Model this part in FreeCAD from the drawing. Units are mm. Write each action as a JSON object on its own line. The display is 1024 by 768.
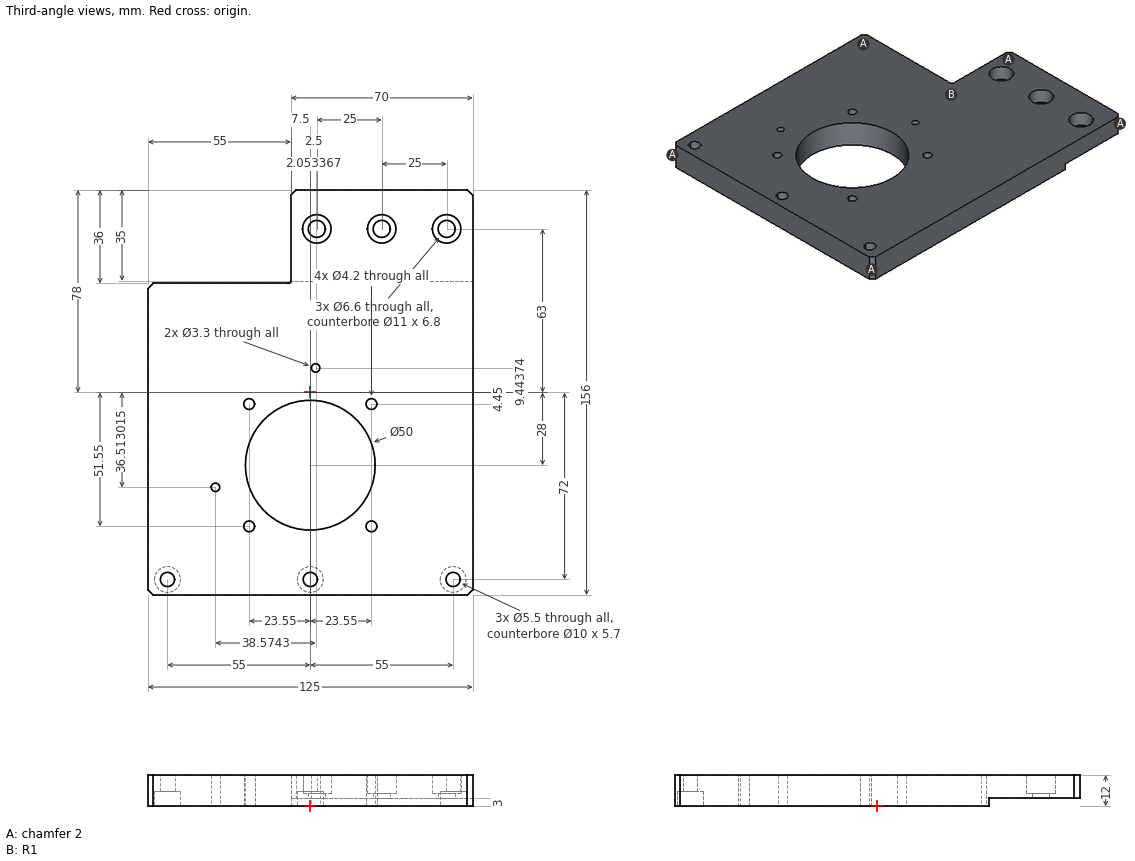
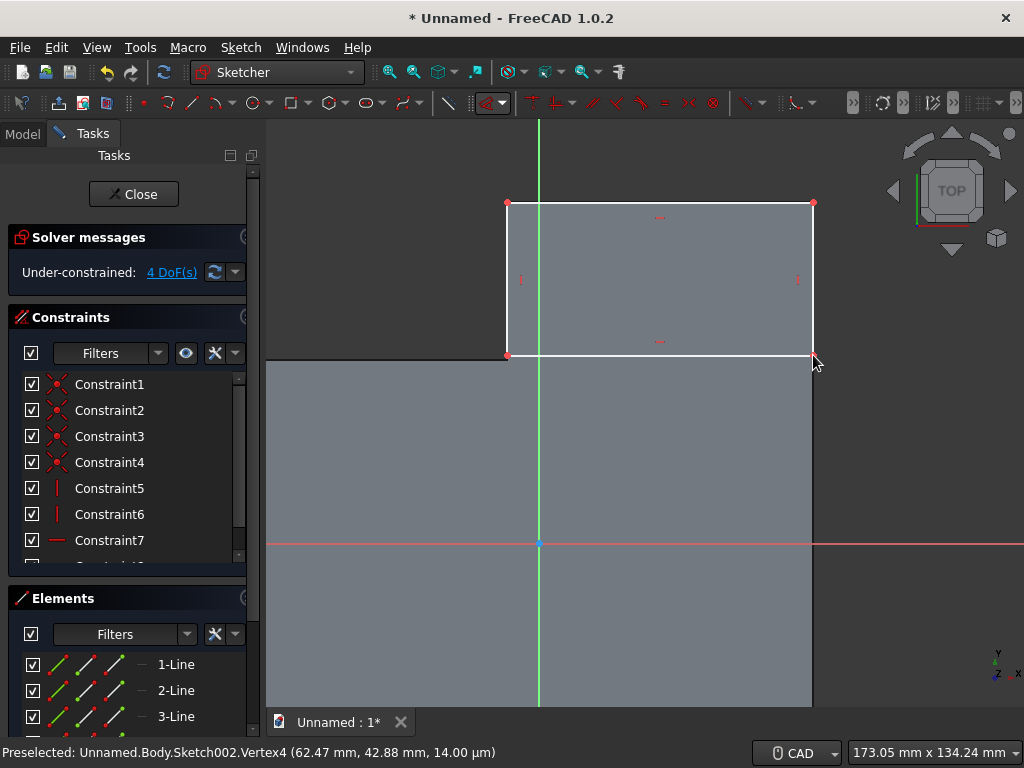
{"action": "left_click", "coordinate": [507, 249]}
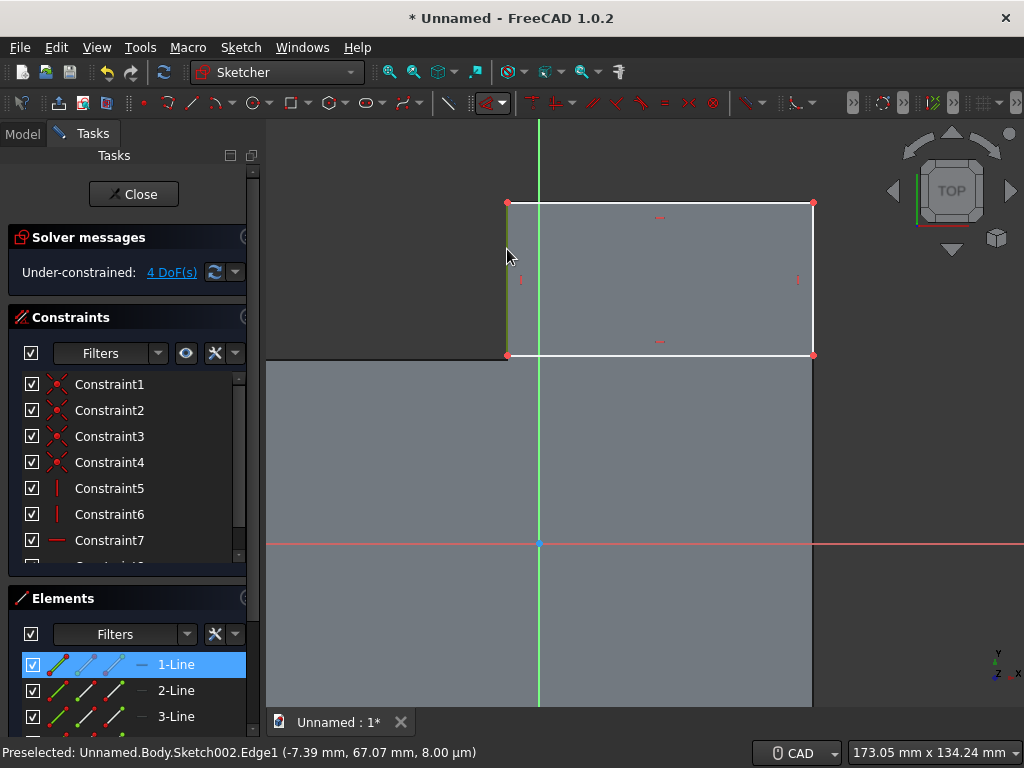
{"action": "left_click", "coordinate": [504, 104]}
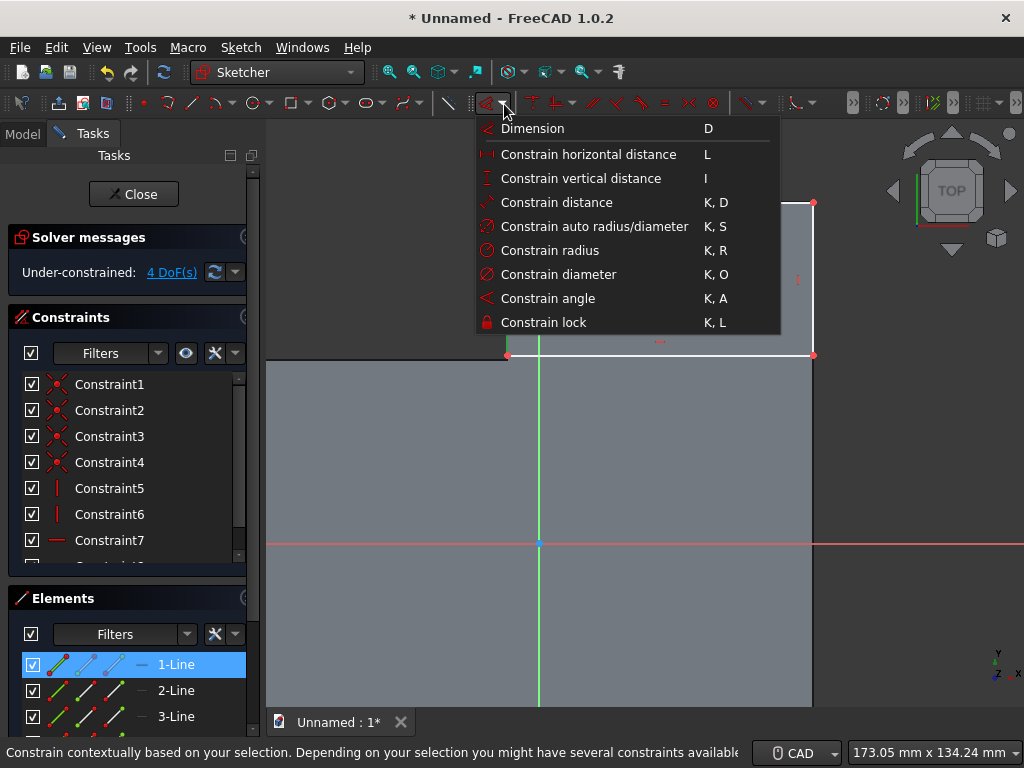
{"action": "left_click", "coordinate": [628, 178]}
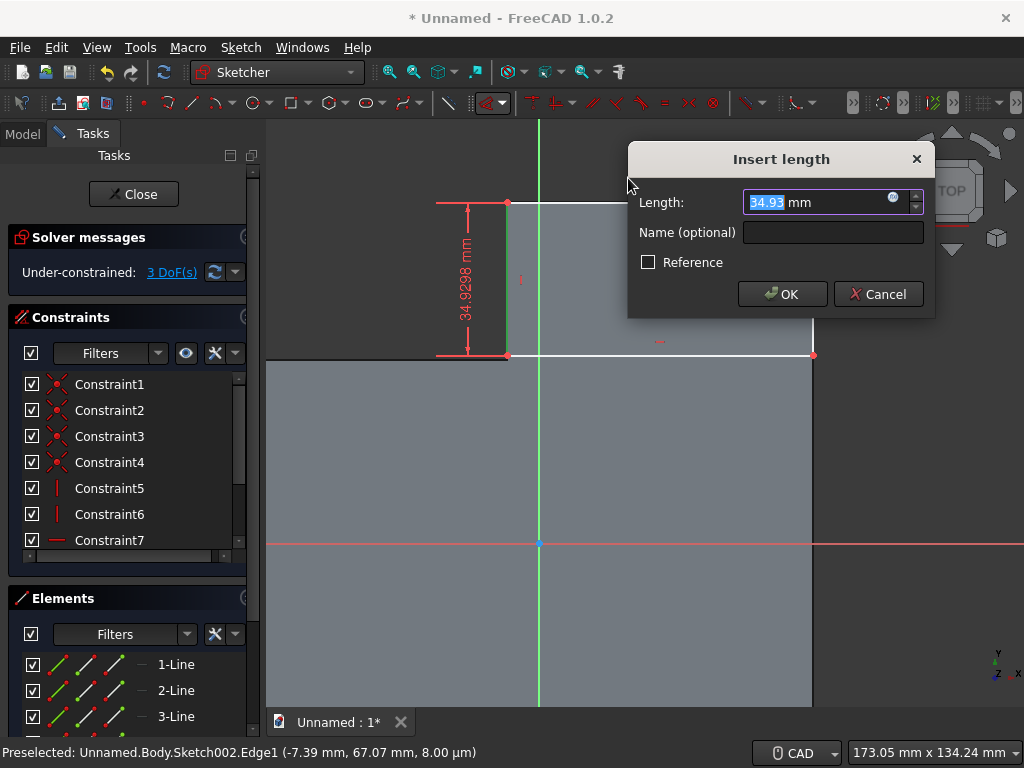
{"action": "type", "text": "35"}
{"action": "key", "text": "Return"}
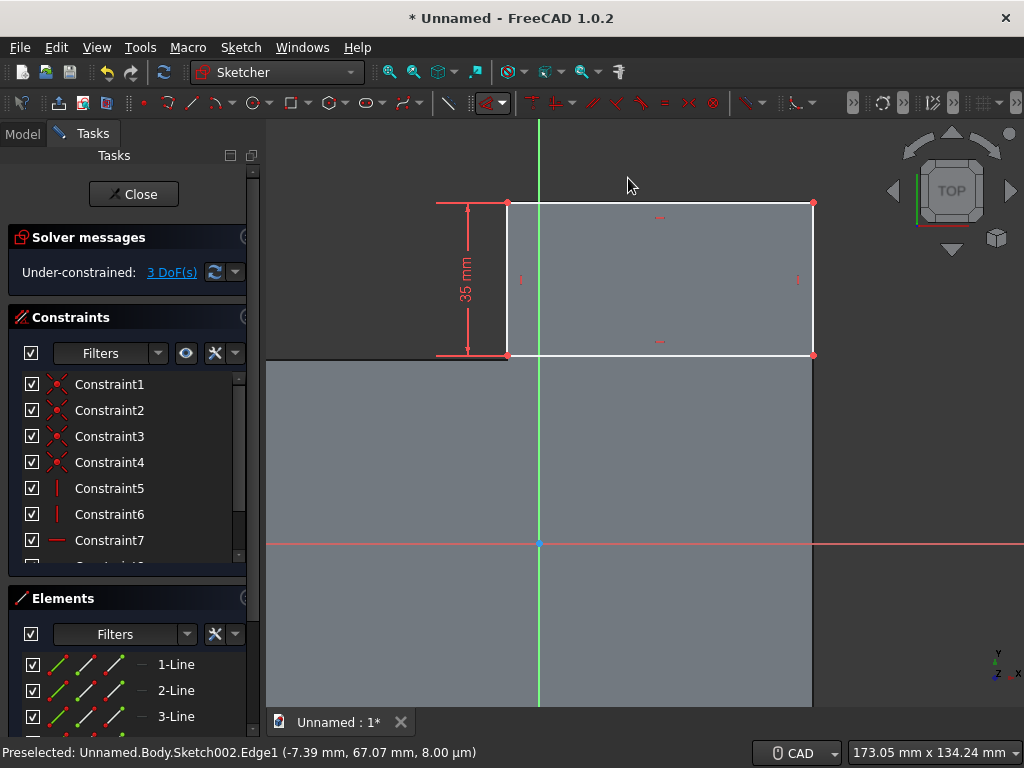
{"action": "left_click", "coordinate": [599, 356]}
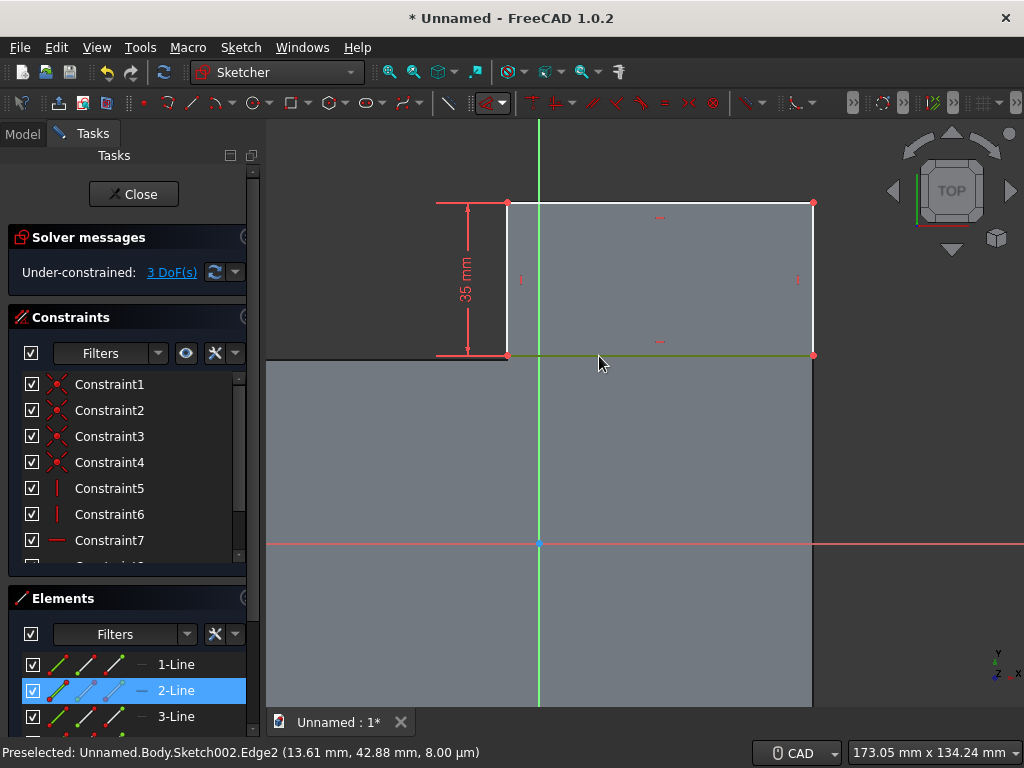
{"action": "key", "text": "l"}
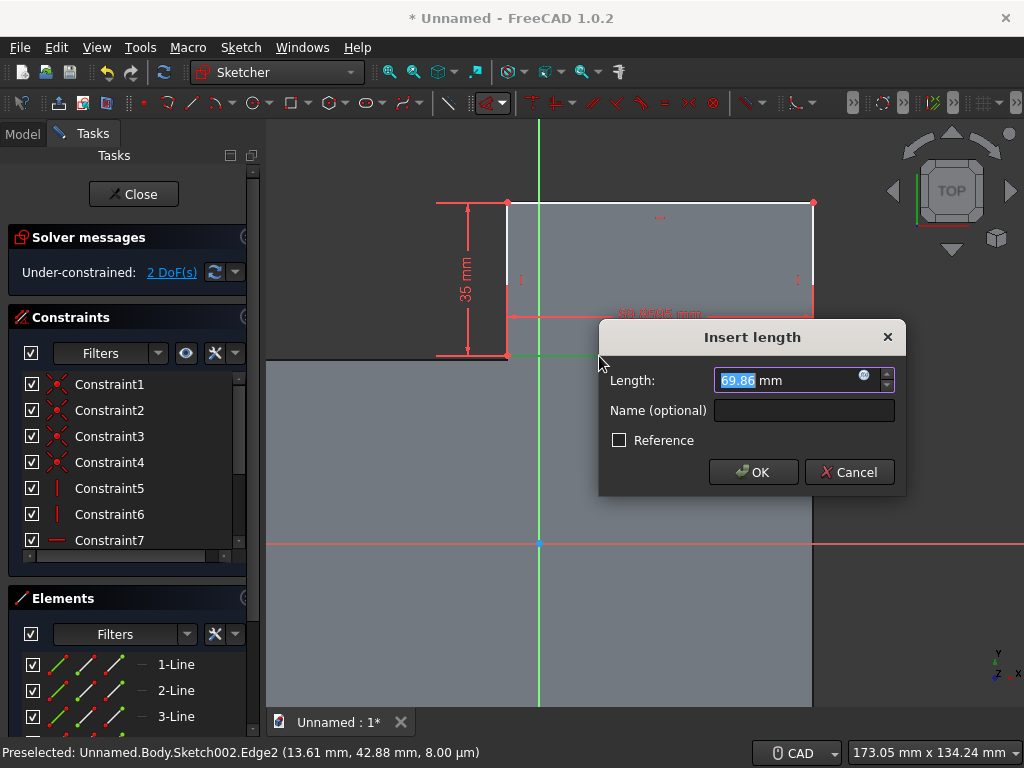
{"action": "type", "text": "70"}
{"action": "key", "text": "Return"}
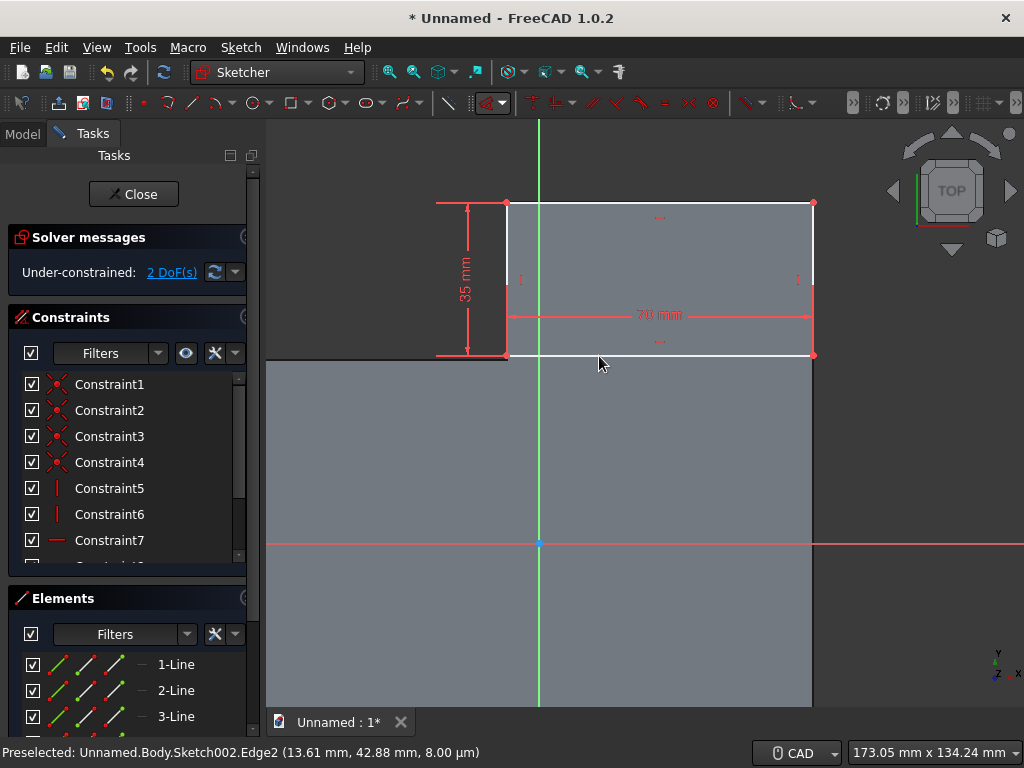
{"action": "left_click", "coordinate": [507, 203]}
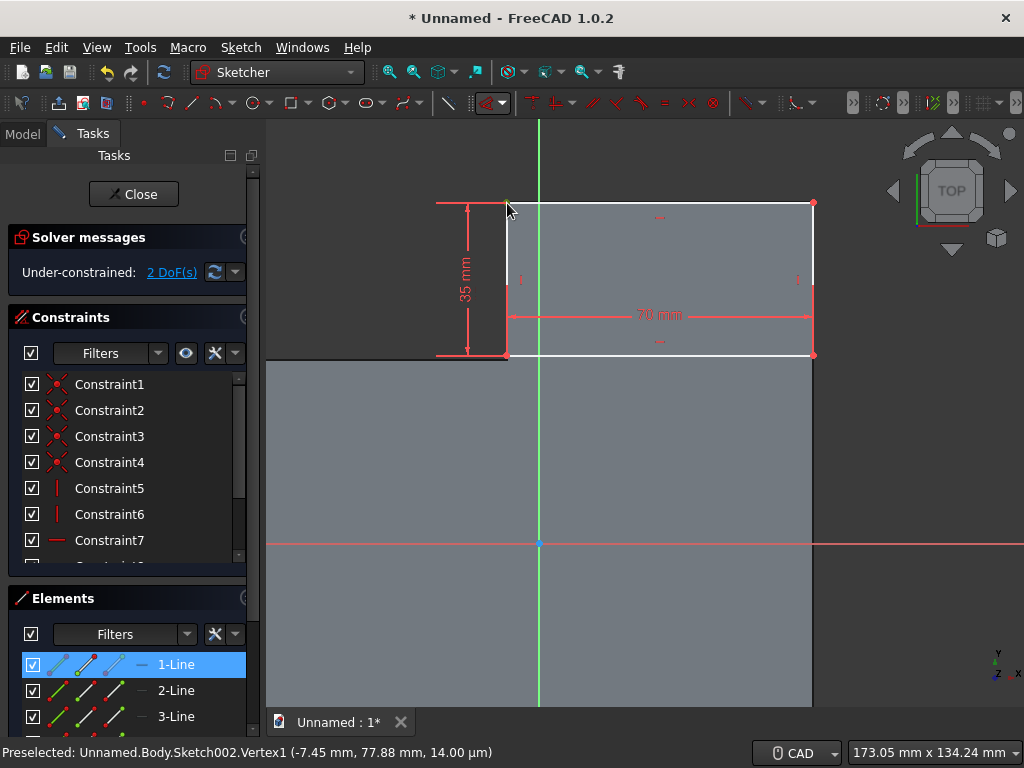
{"action": "left_click", "coordinate": [504, 104]}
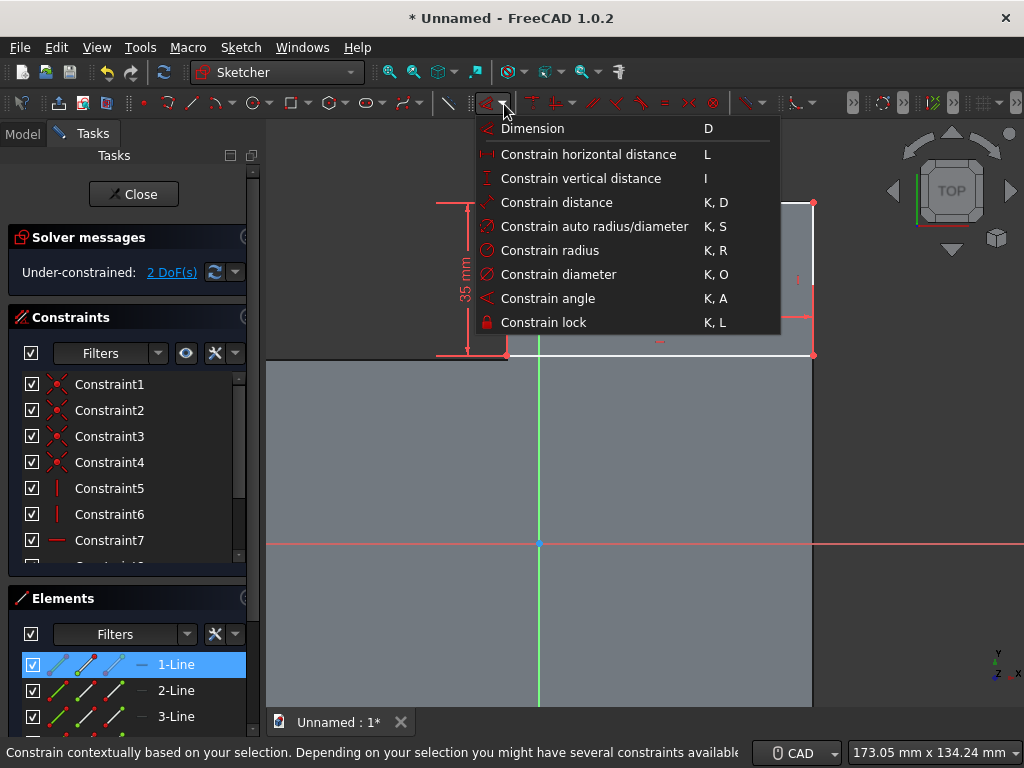
{"action": "left_click", "coordinate": [628, 178]}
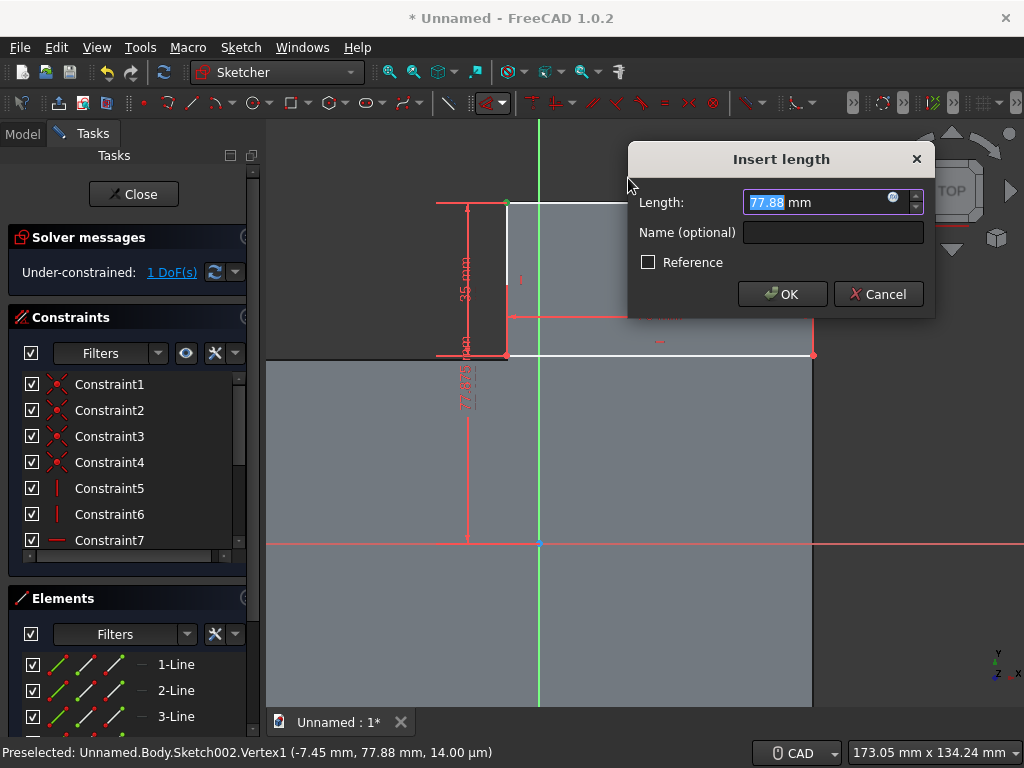
{"action": "type", "text": "78"}
{"action": "key", "text": "Return"}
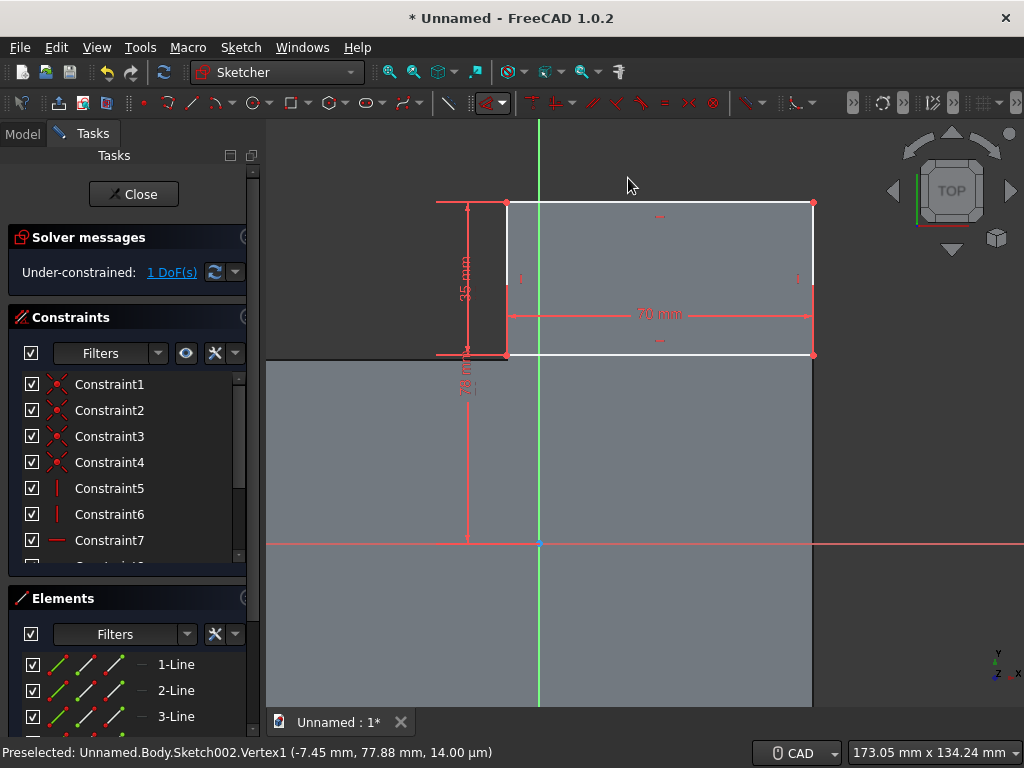
{"action": "left_click", "coordinate": [507, 202]}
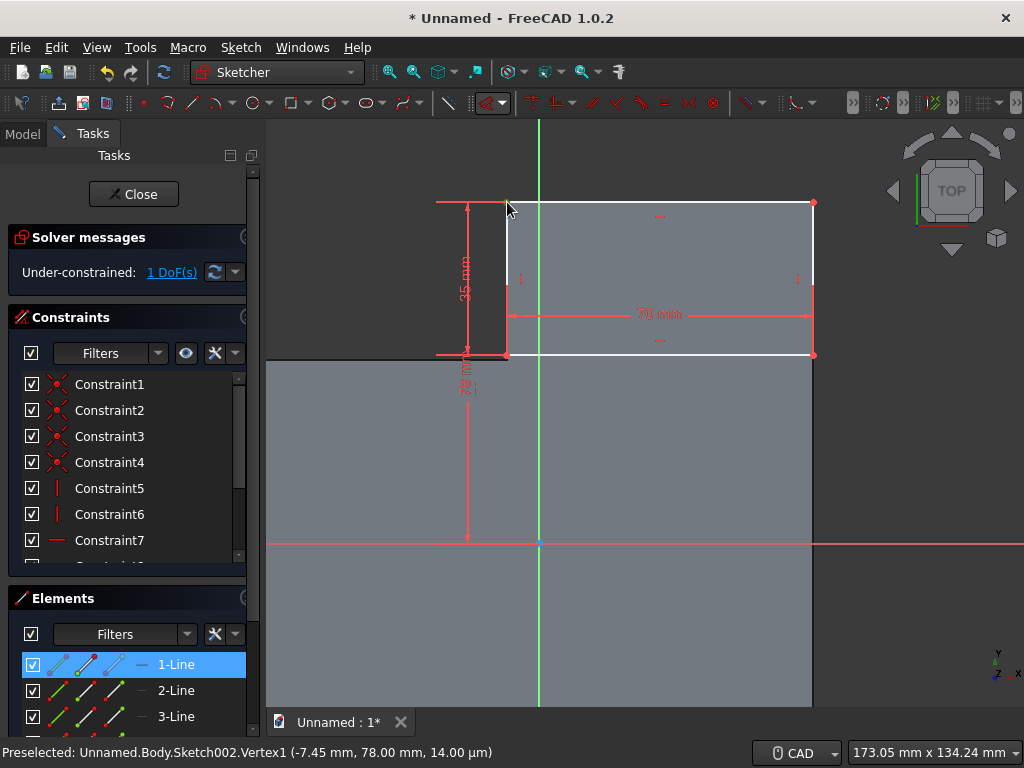
{"action": "key", "text": "l"}